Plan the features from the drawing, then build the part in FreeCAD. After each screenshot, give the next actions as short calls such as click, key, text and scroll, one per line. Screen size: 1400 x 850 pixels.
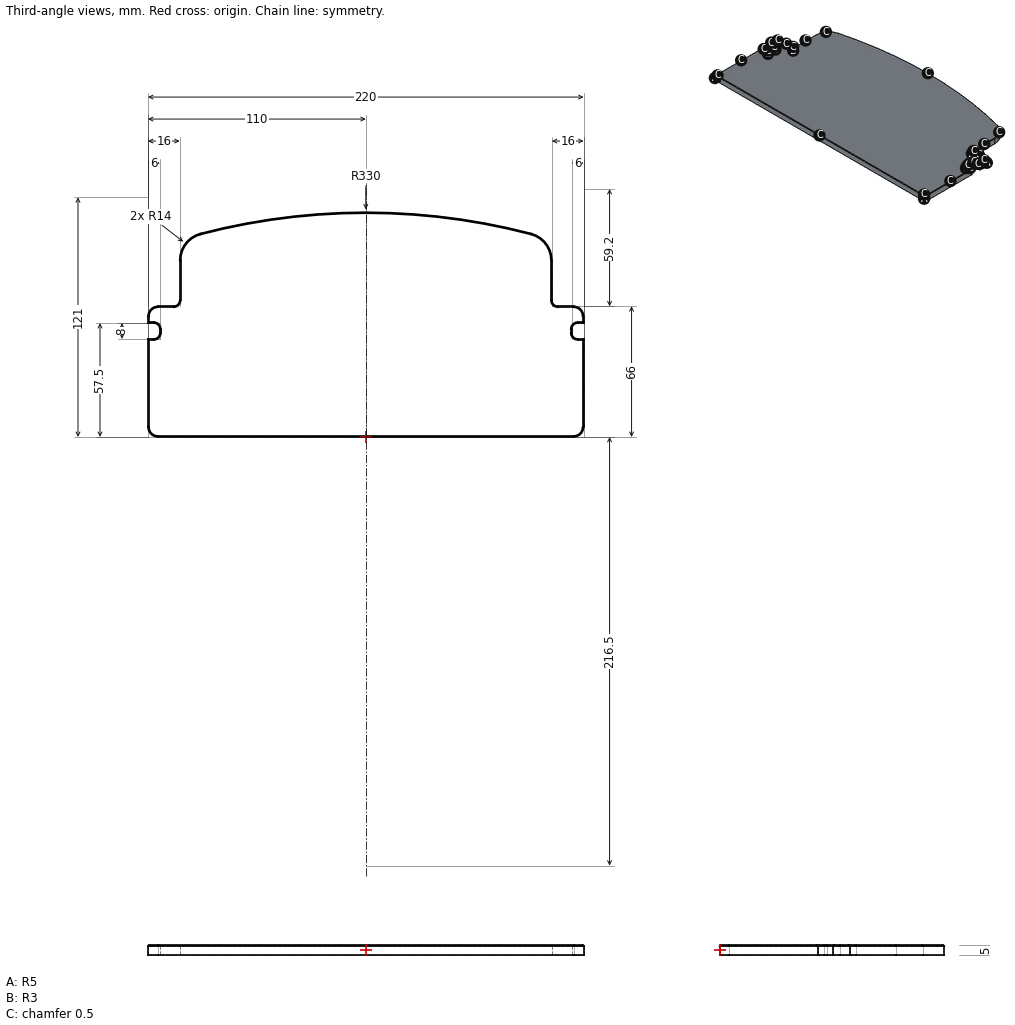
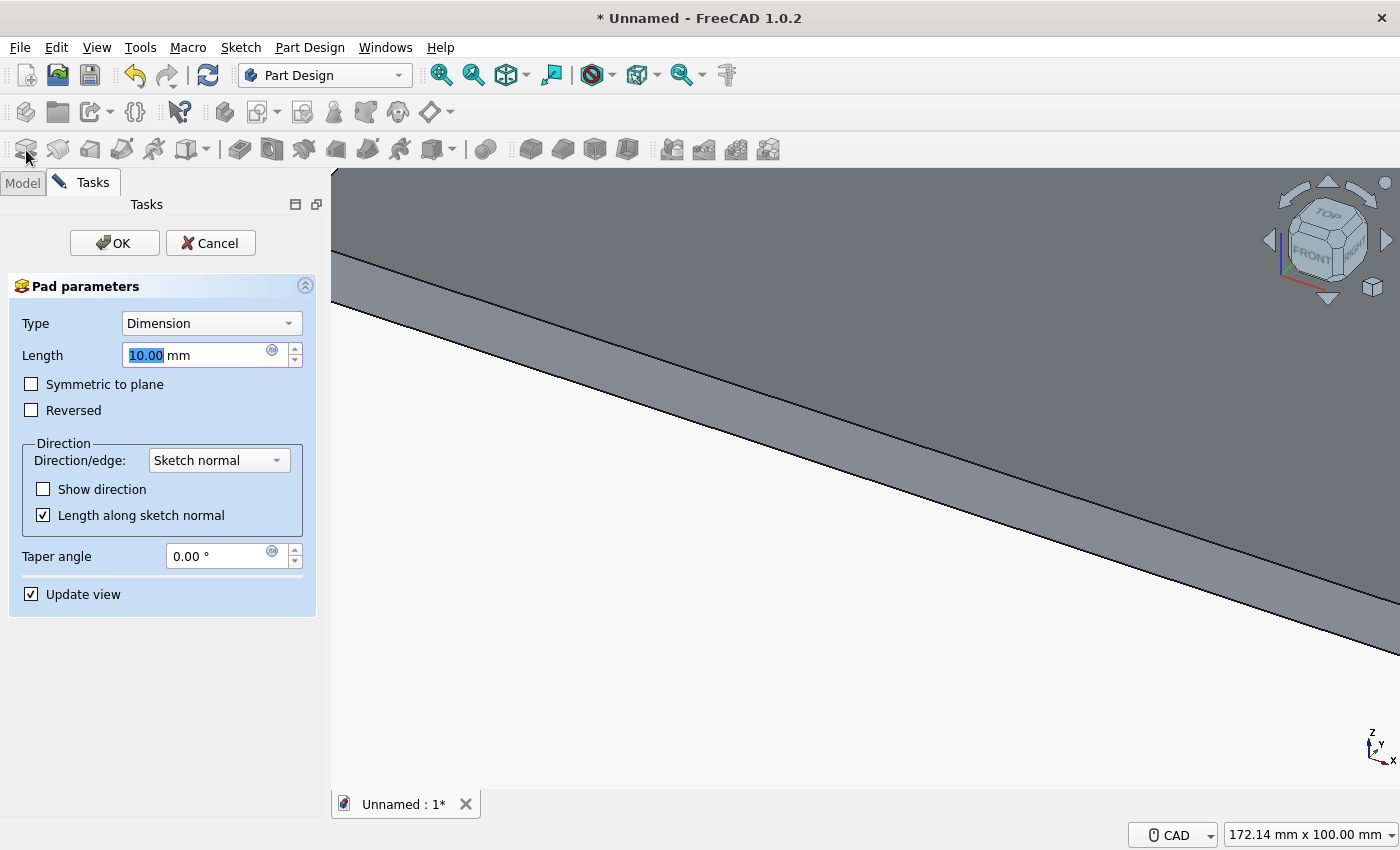
text(5)
key(Tab)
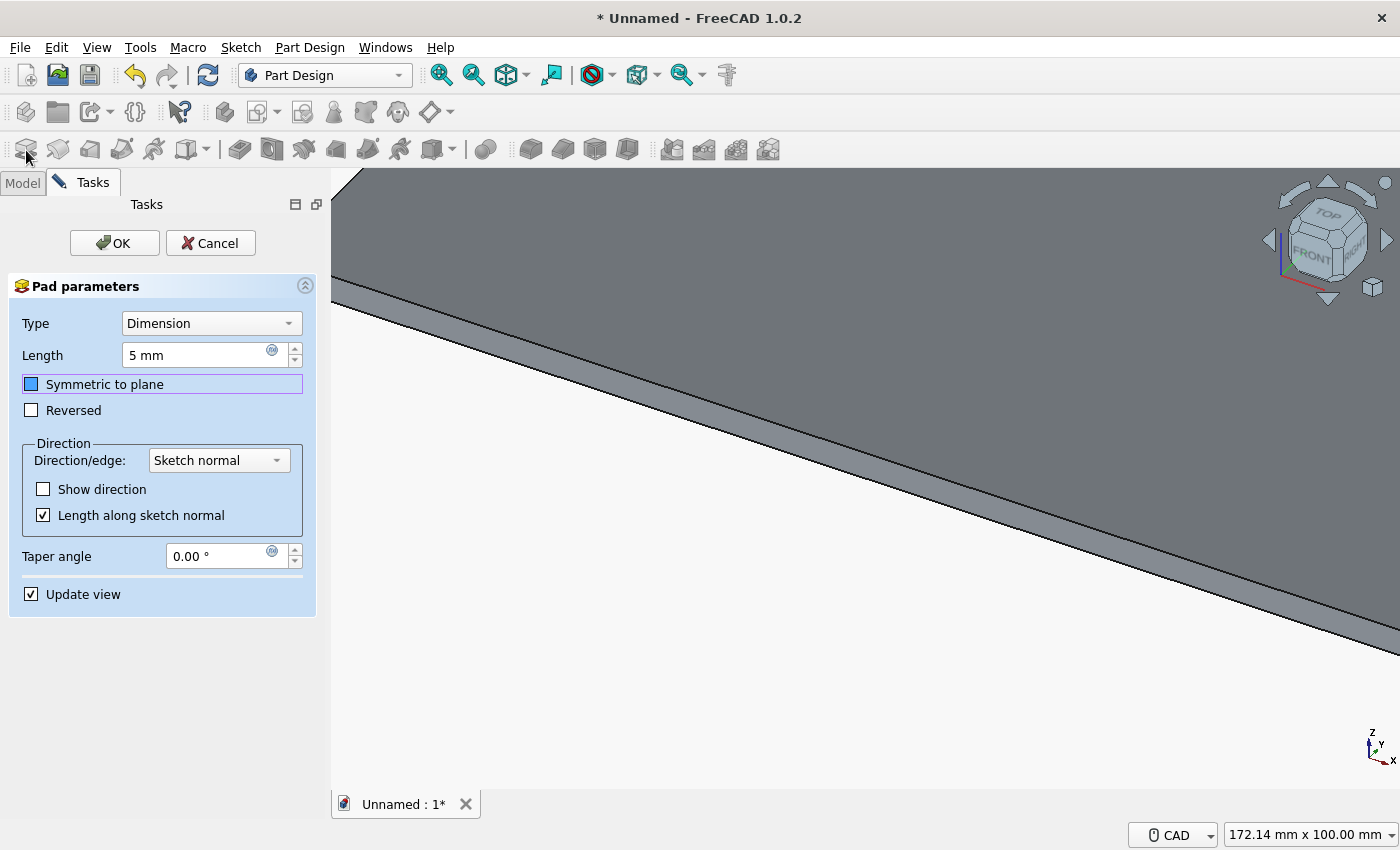
click(30, 384)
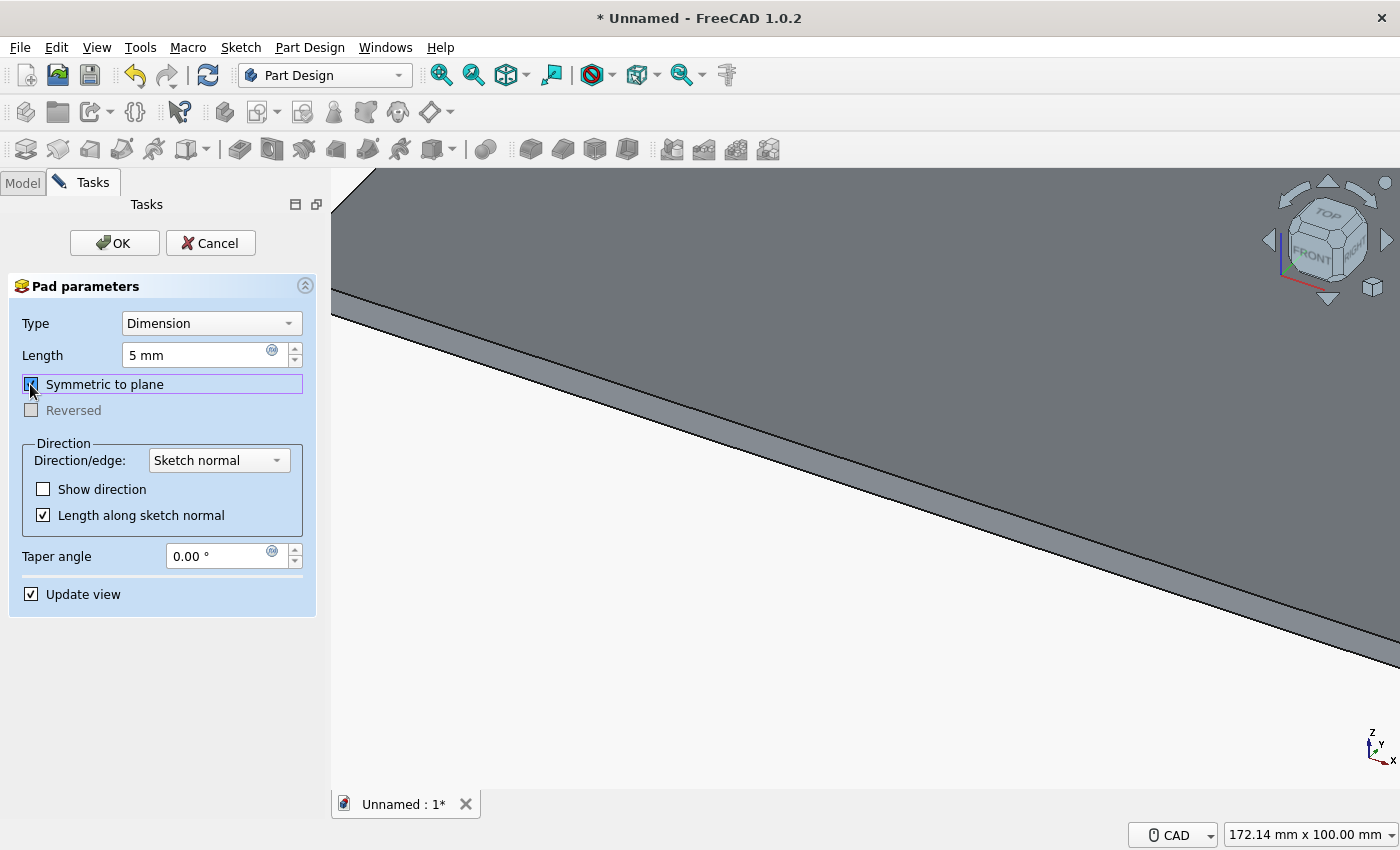
click(115, 243)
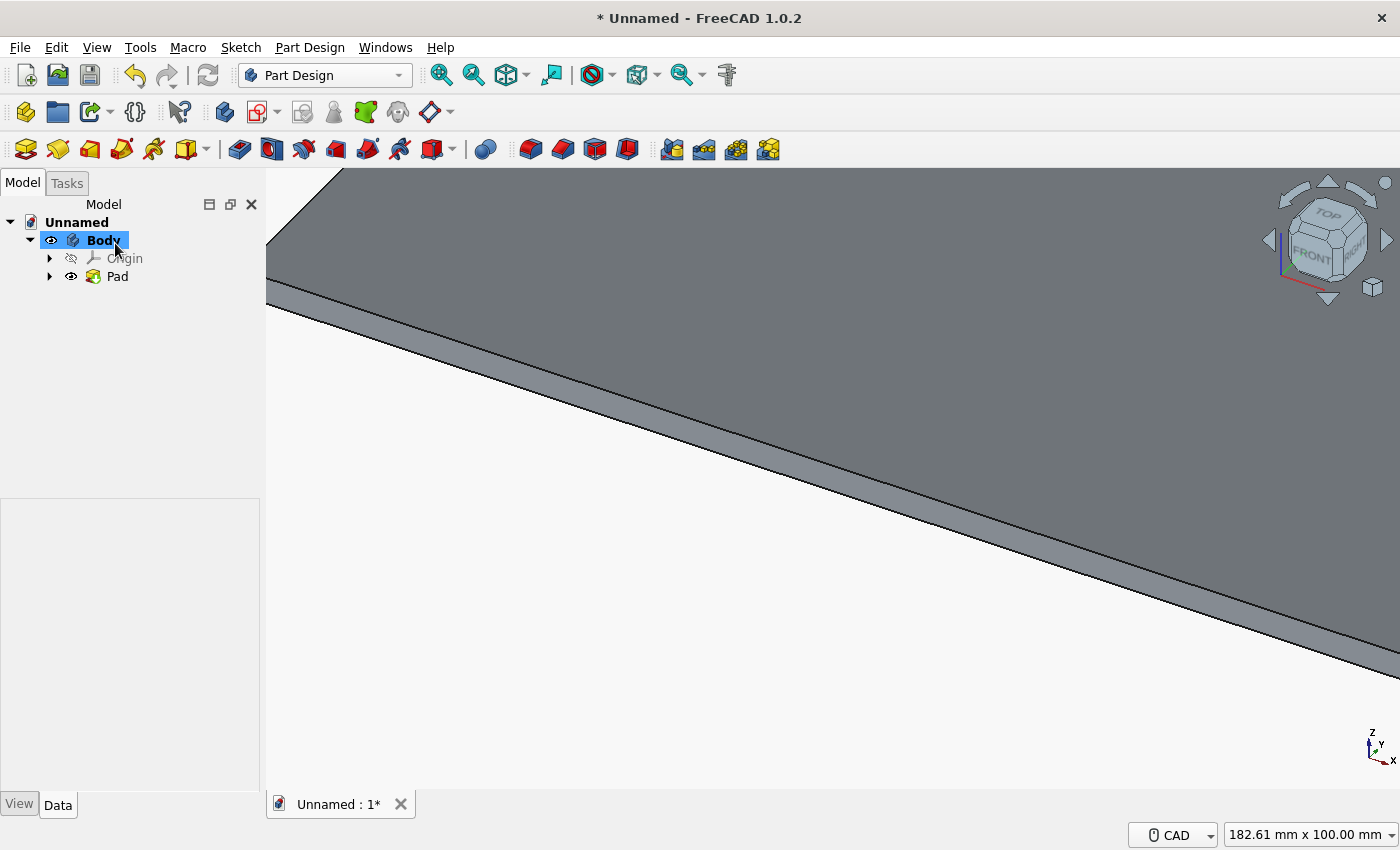
key(v)
key(f)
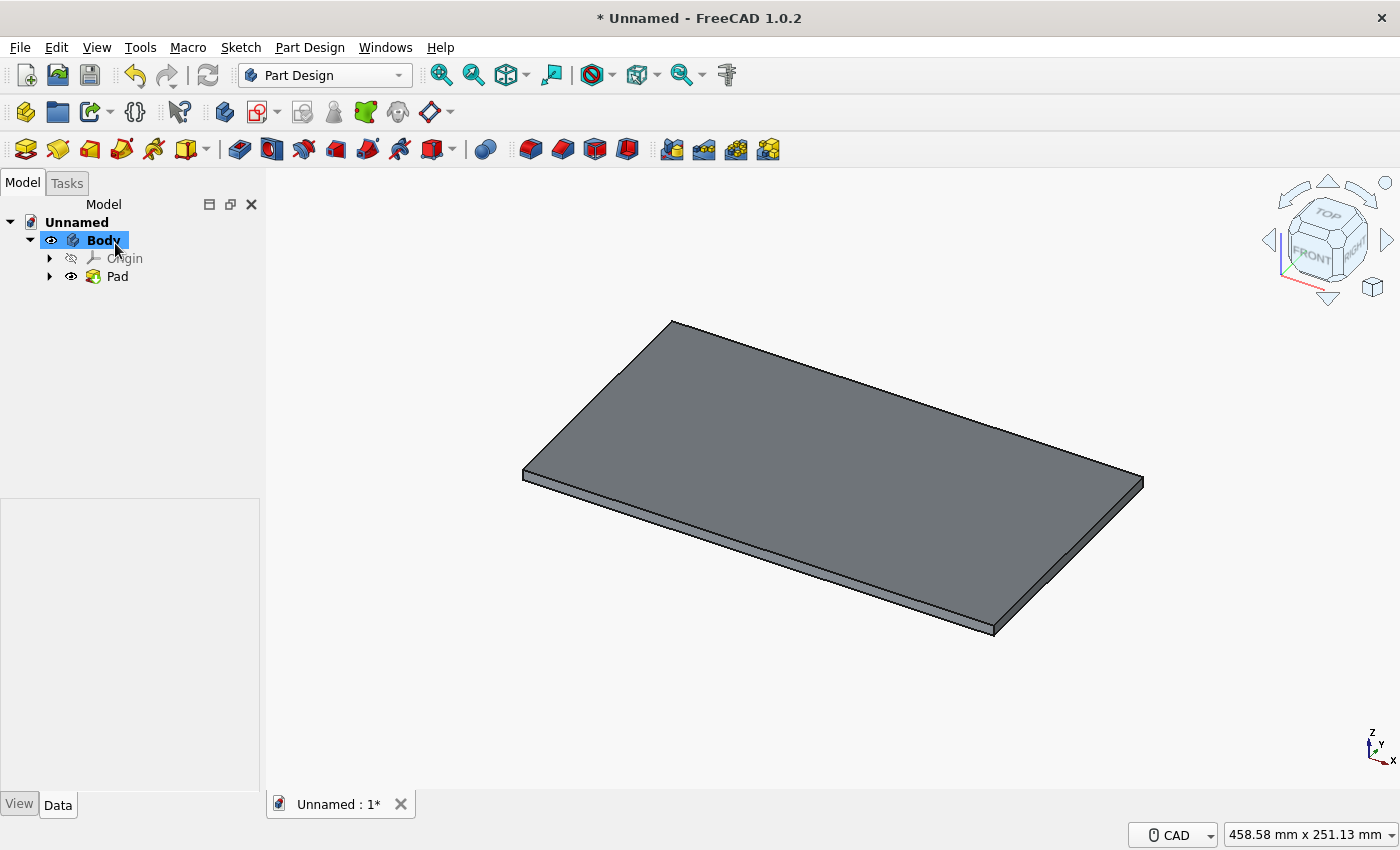
click(900, 495)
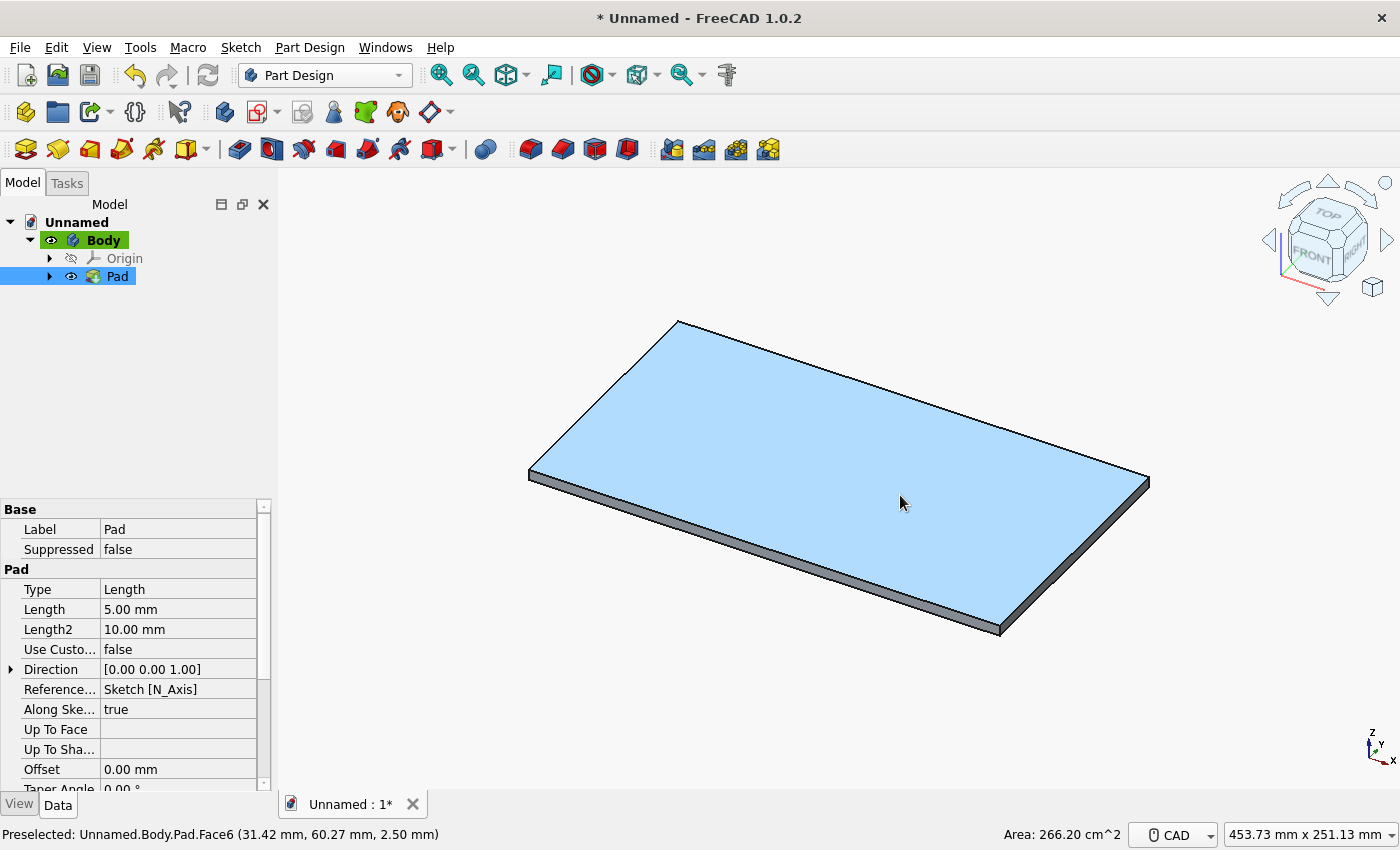
click(258, 112)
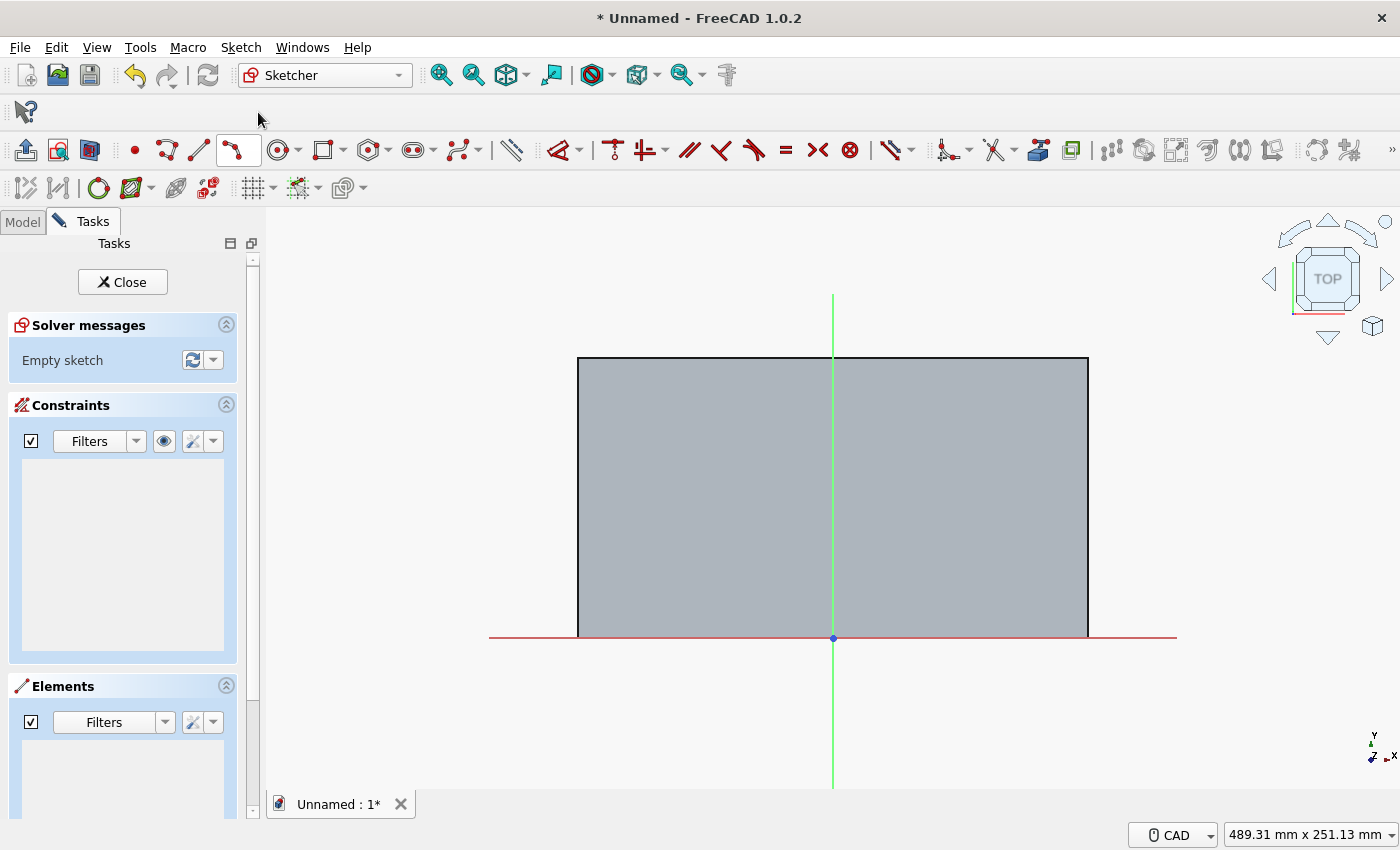
click(168, 150)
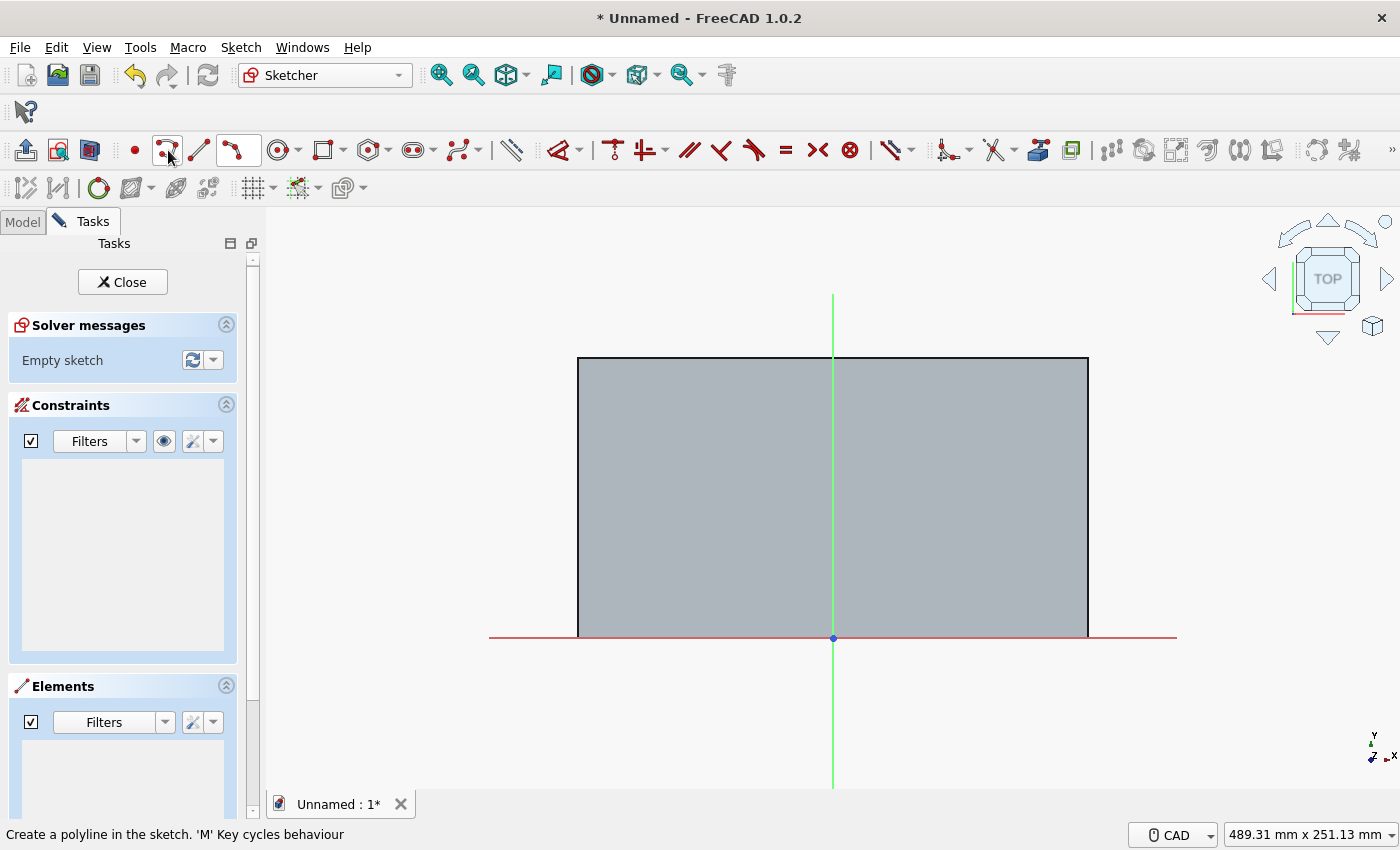
click(1051, 431)
click(1051, 485)
click(1088, 485)
click(1088, 348)
click(578, 348)
click(578, 485)
click(615, 485)
click(615, 431)
right_click(615, 431)